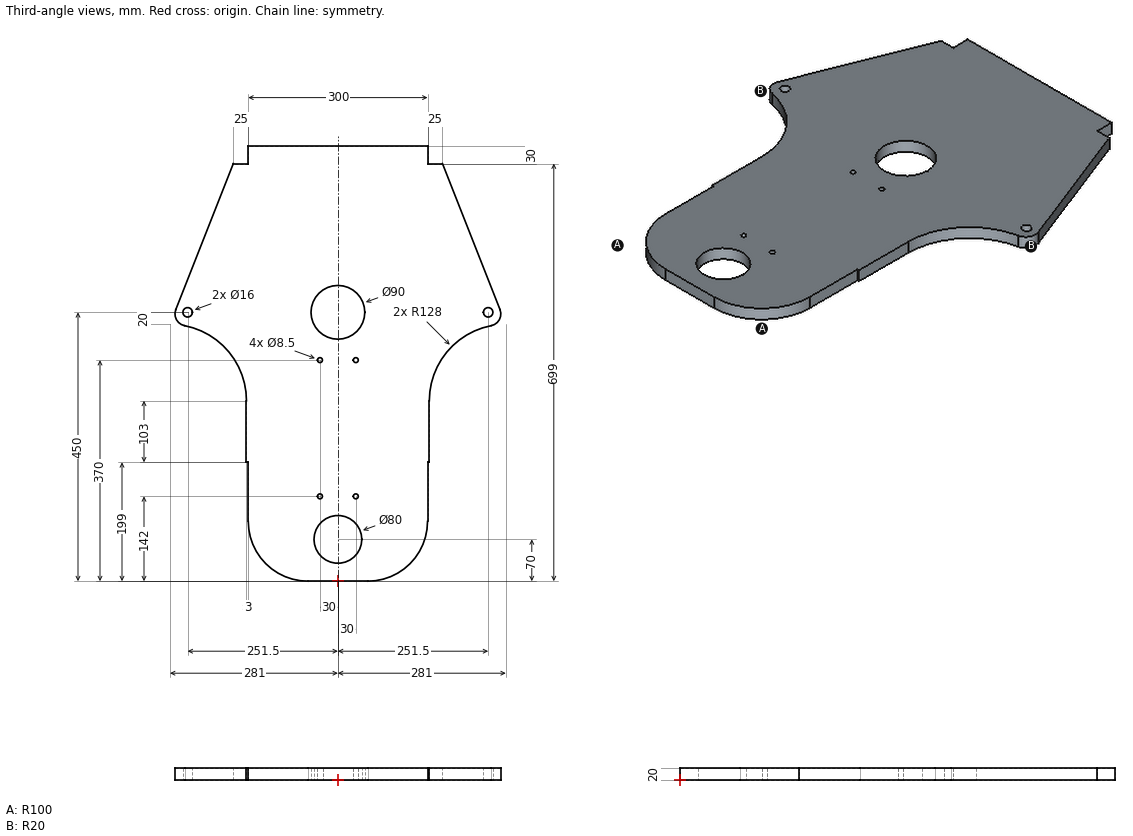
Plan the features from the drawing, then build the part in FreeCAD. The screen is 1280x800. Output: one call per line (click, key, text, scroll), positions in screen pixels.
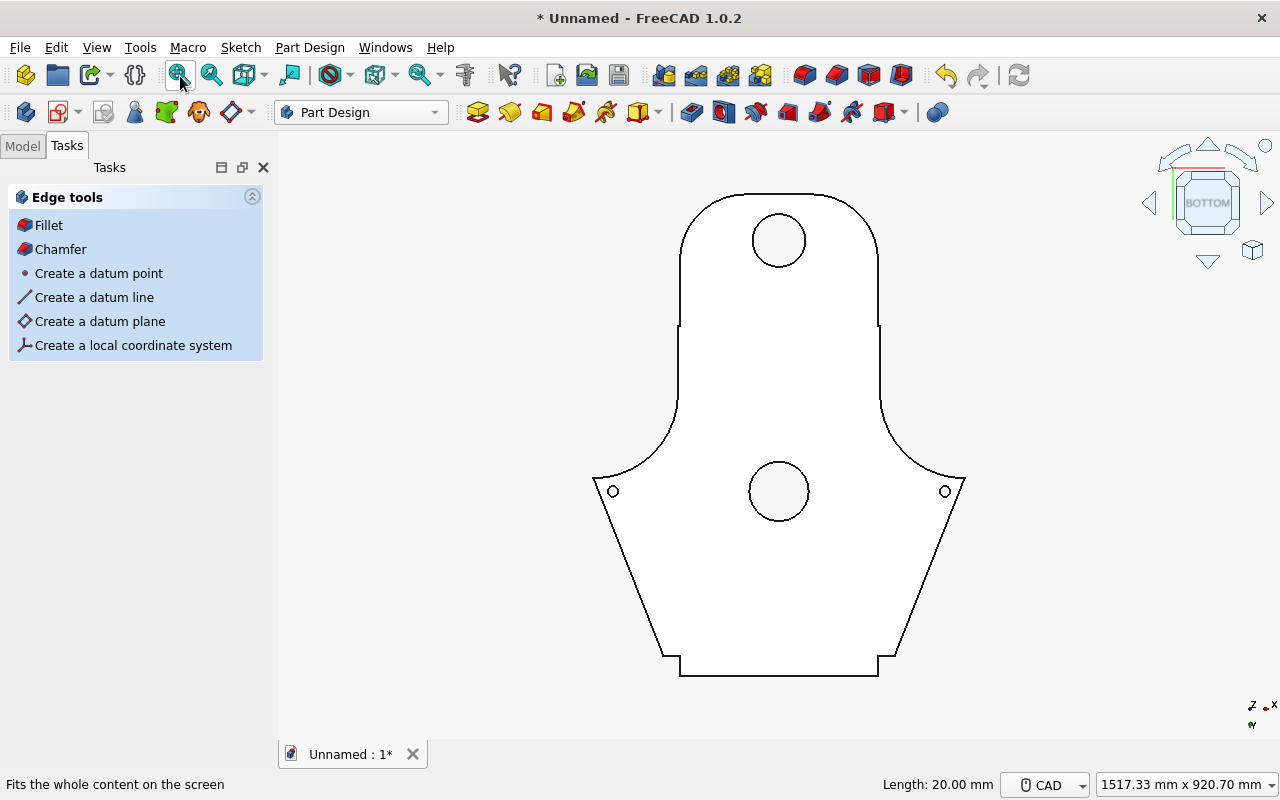
scroll(593, 477, up, 6)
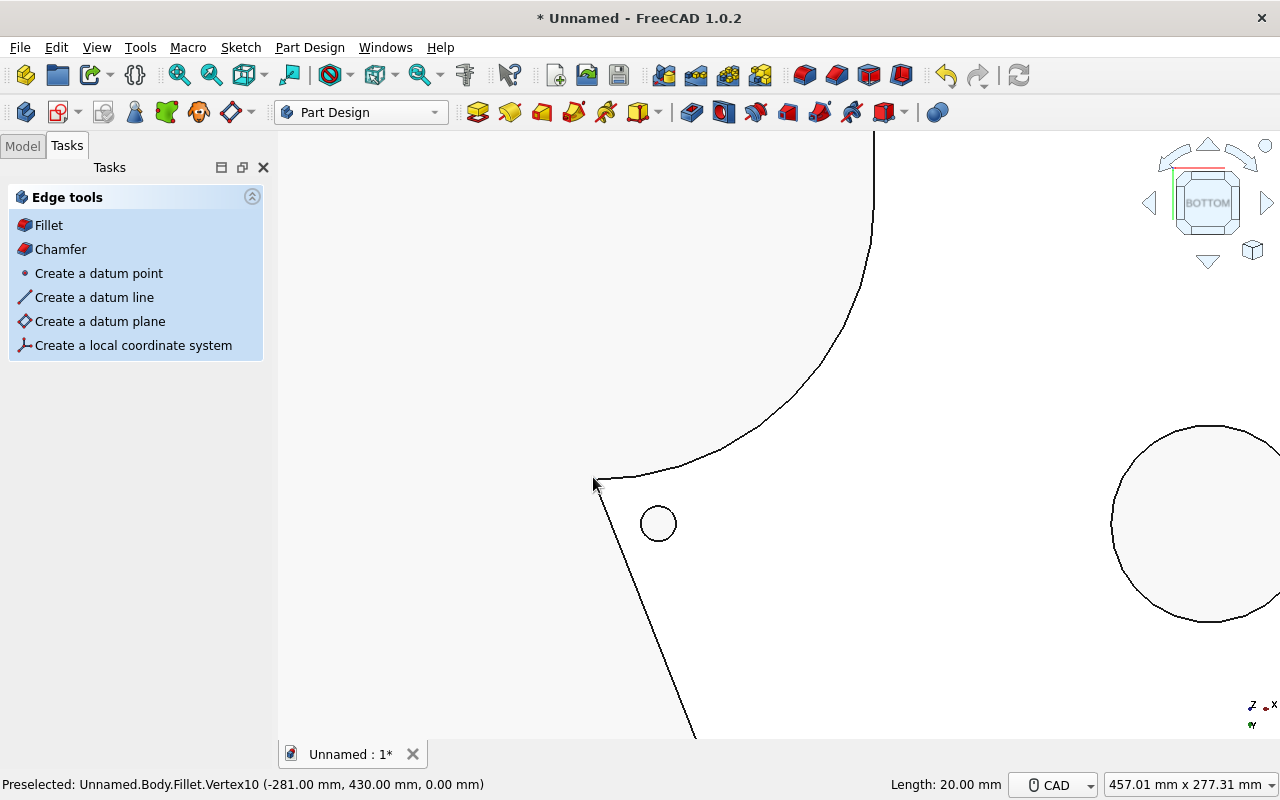
click(180, 76)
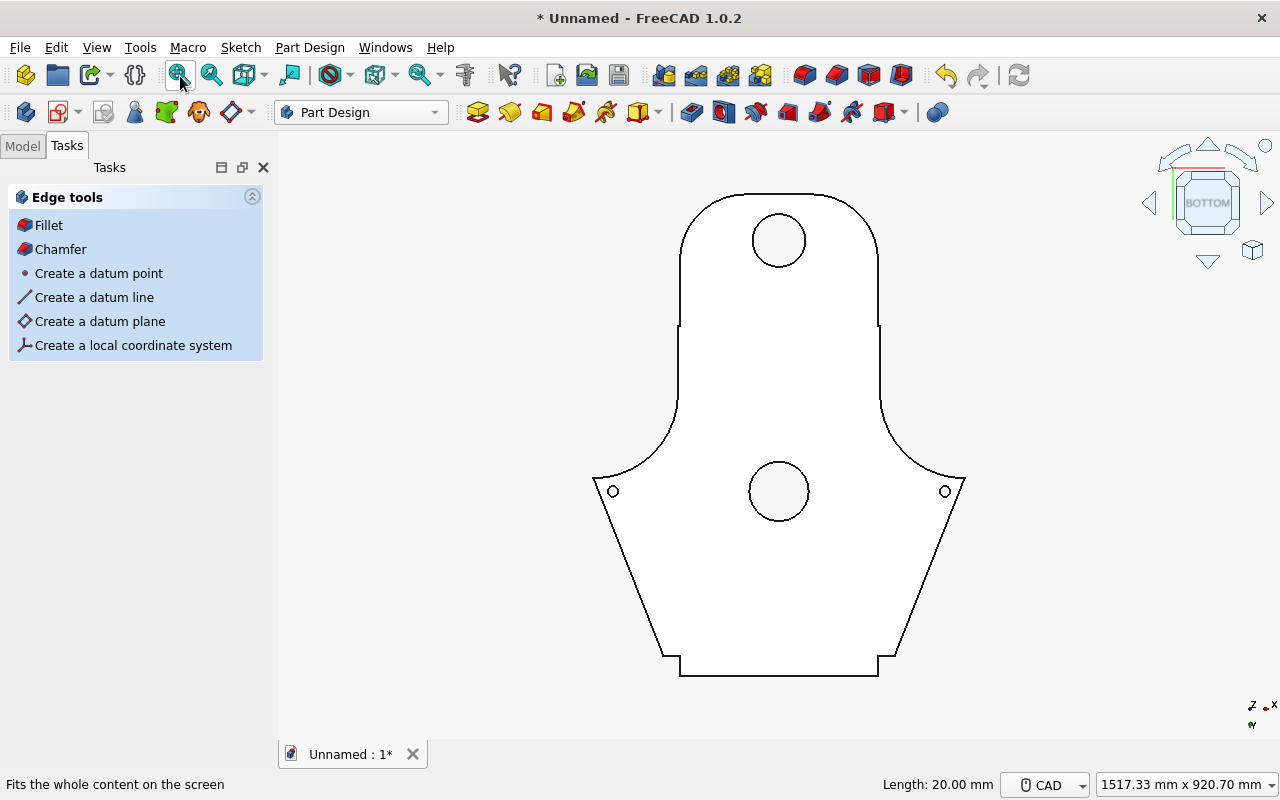
key(4)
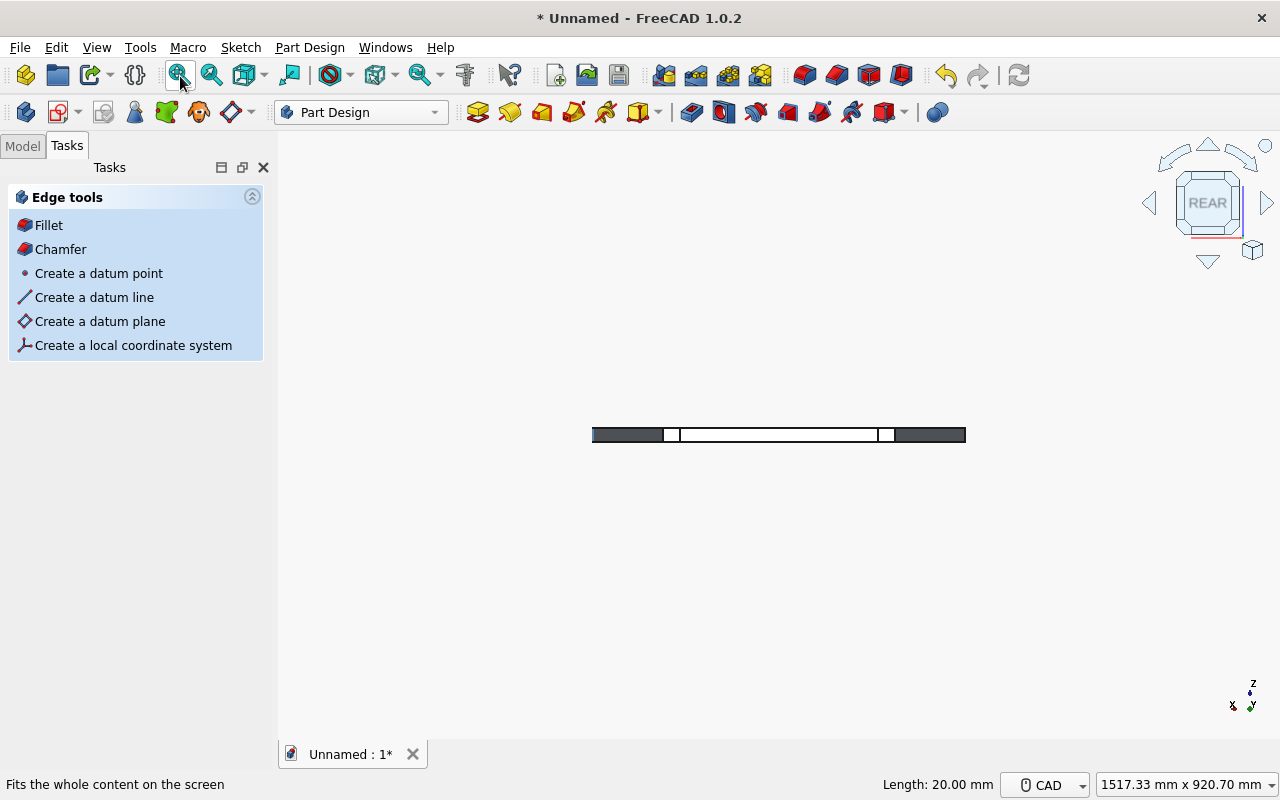
click(180, 76)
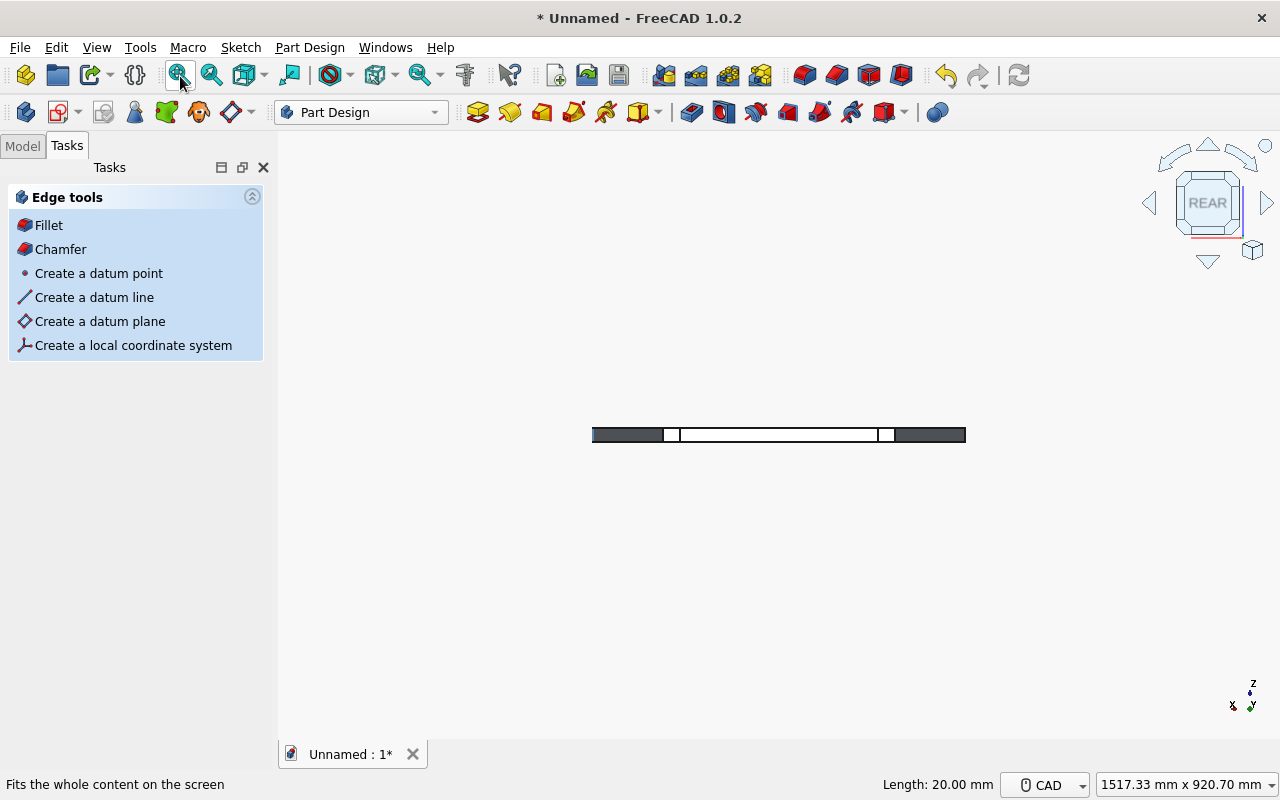
scroll(965, 434, up, 6)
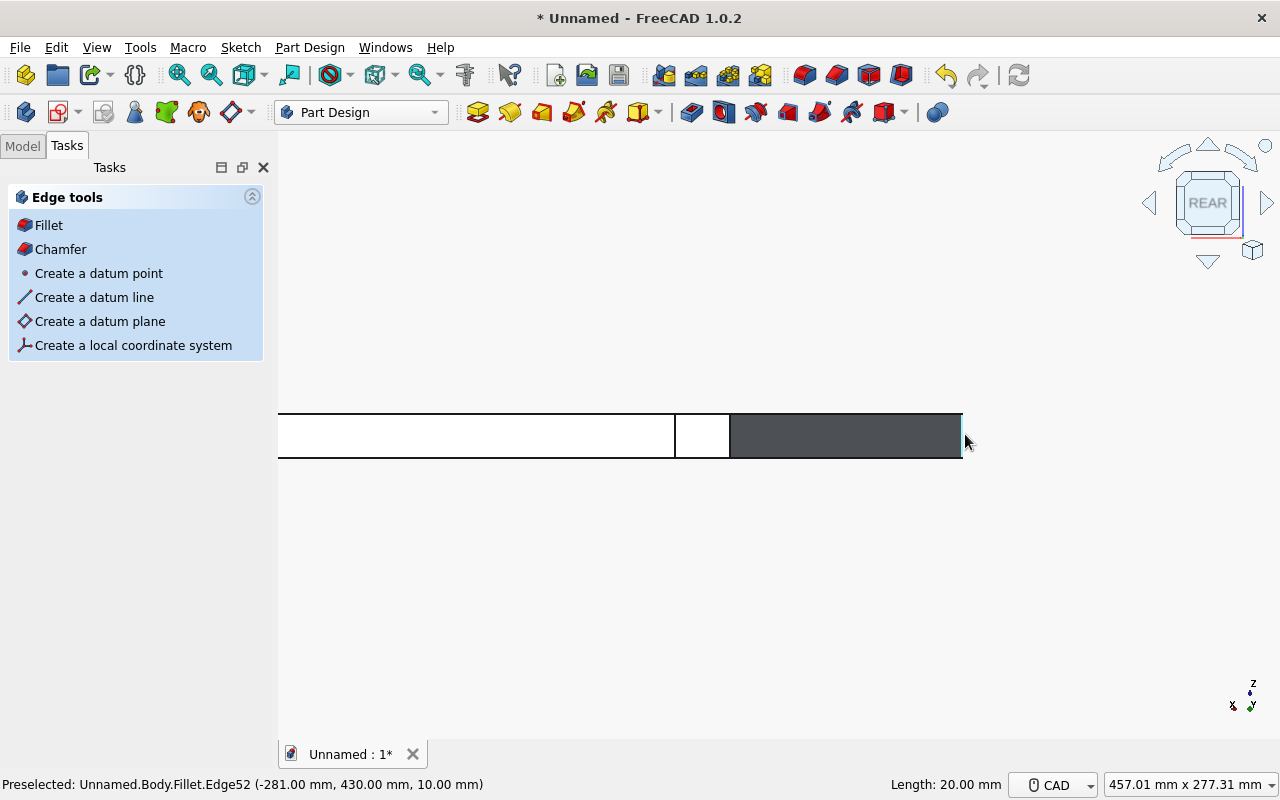
click(180, 76)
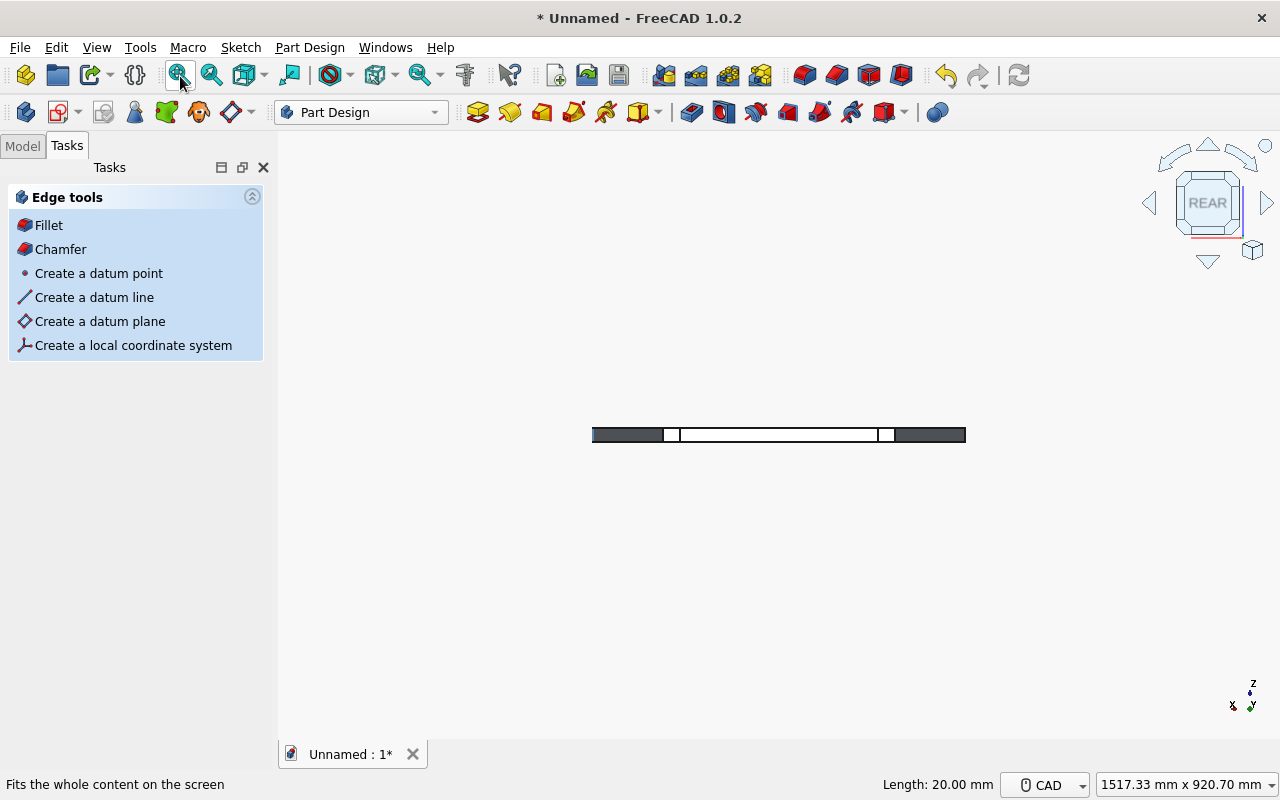
key(6)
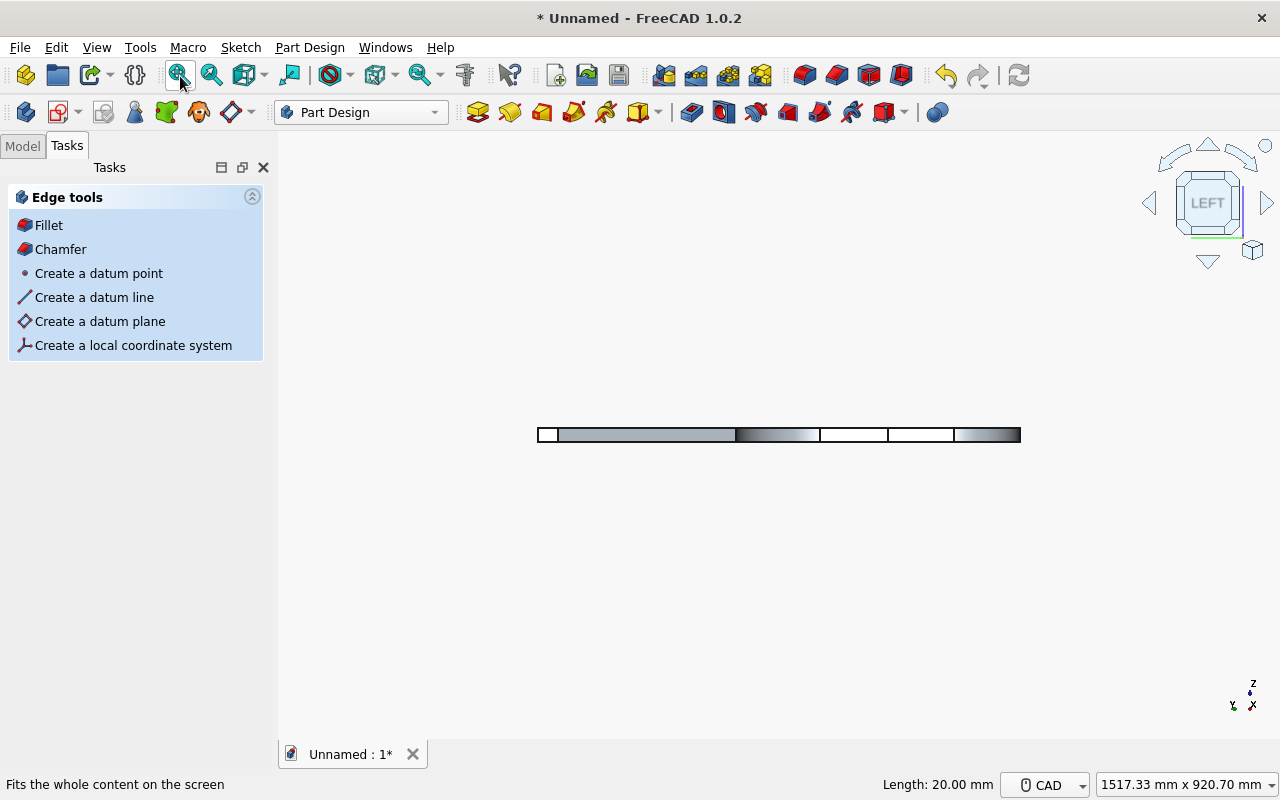
click(736, 434, ctrl)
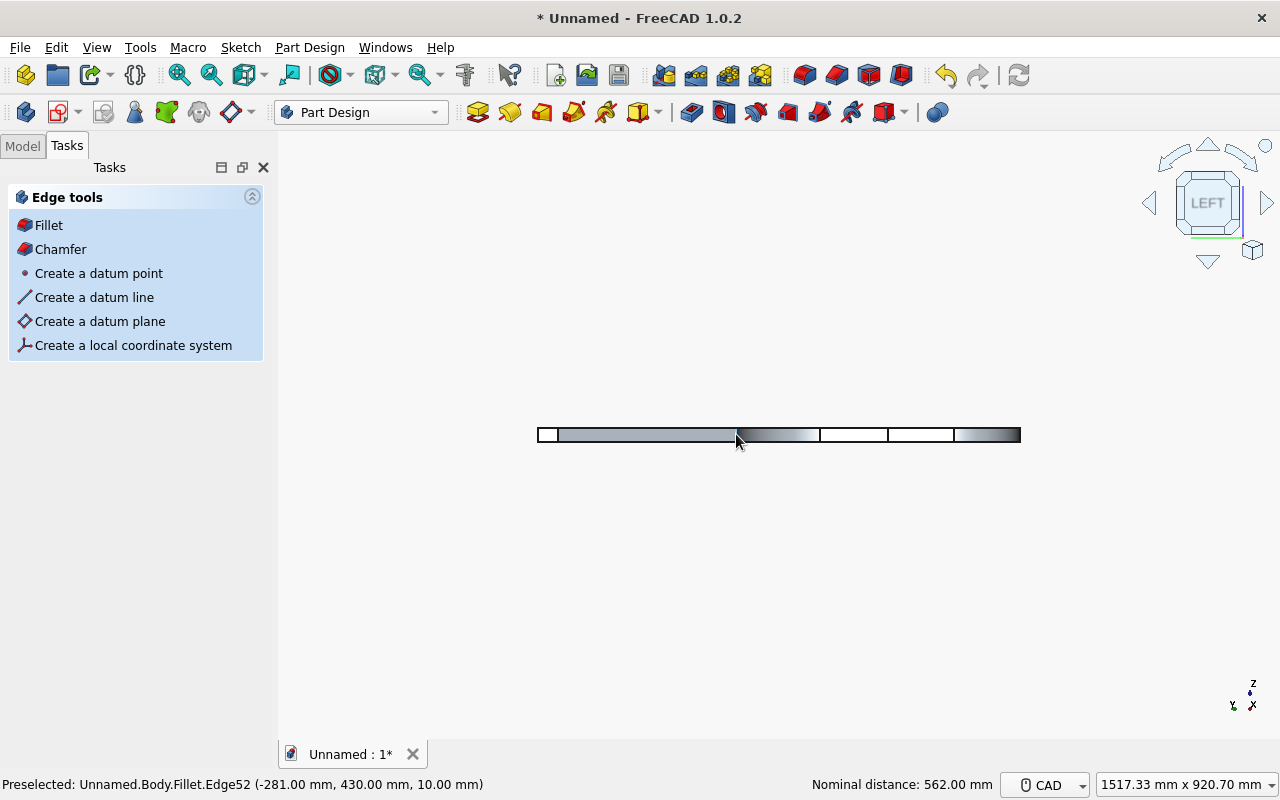
click(806, 76)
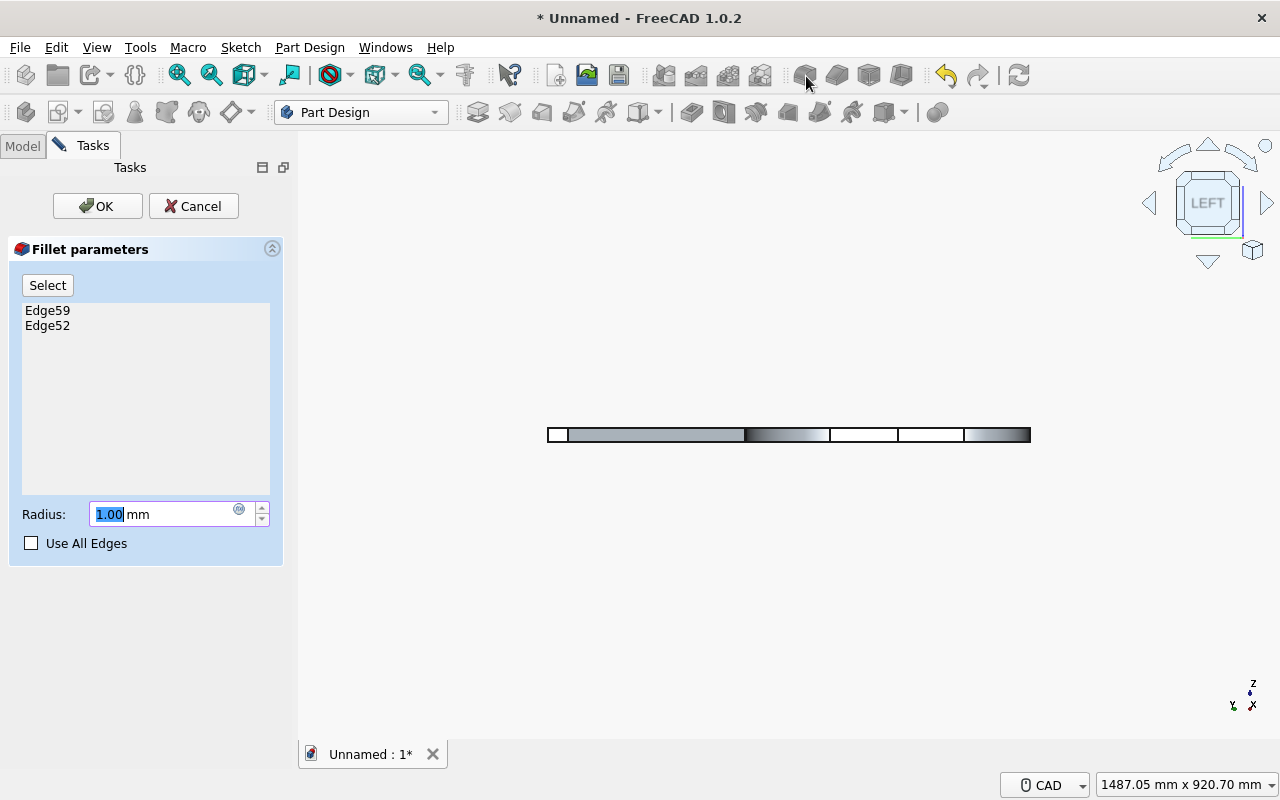
text(20)
key(Tab)